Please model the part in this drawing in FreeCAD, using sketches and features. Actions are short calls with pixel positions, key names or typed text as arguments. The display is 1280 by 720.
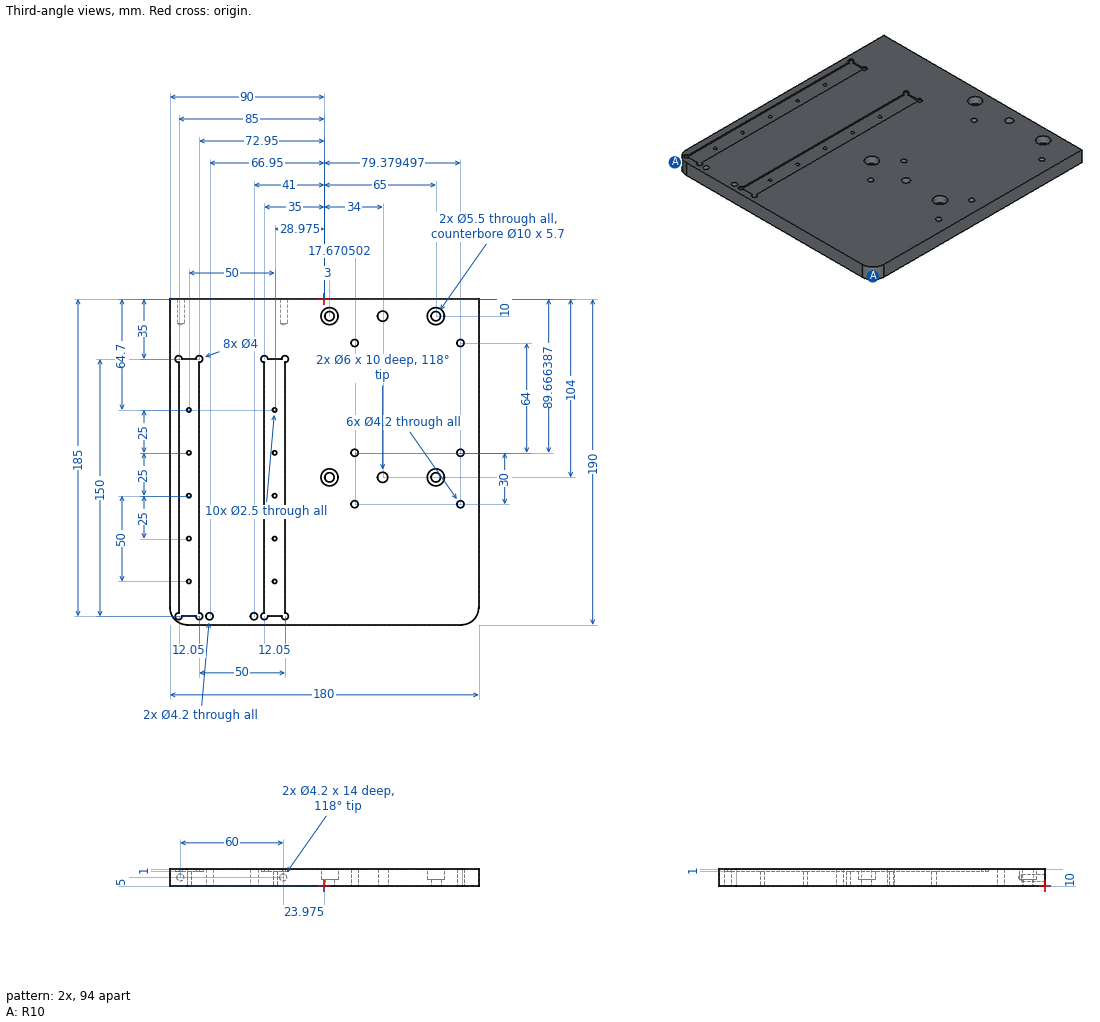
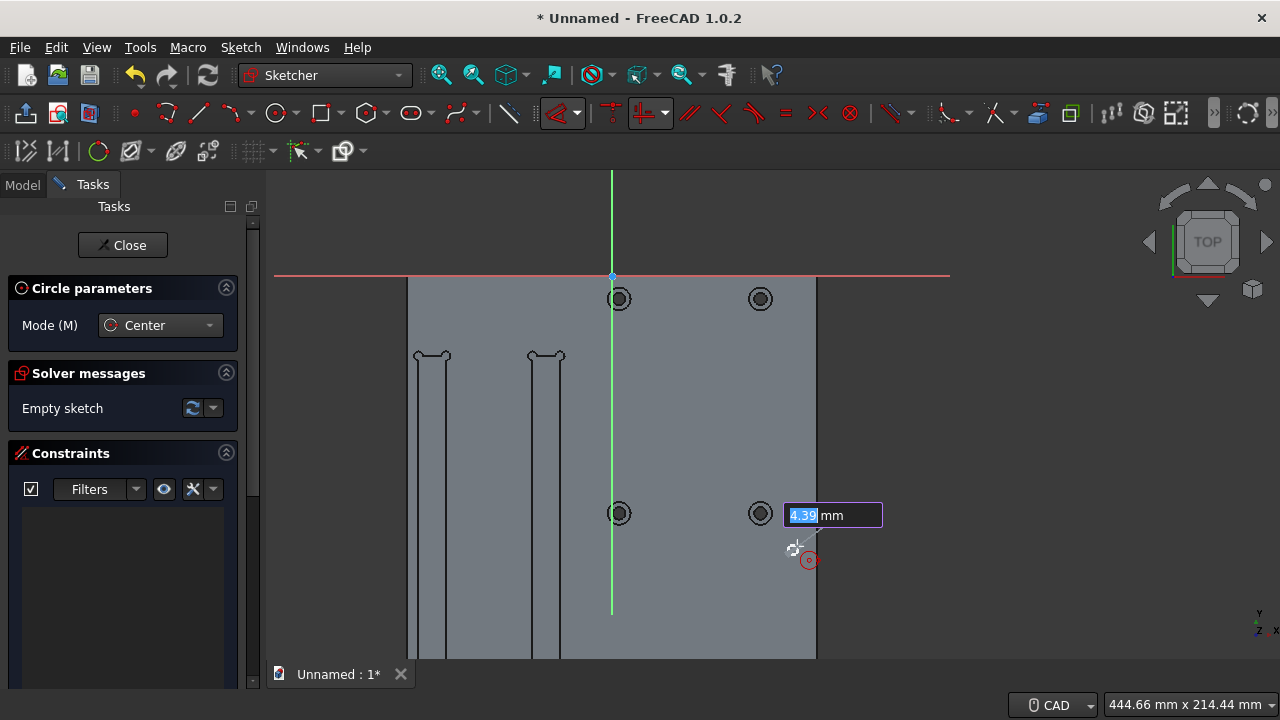
text(4.2)
key(Return)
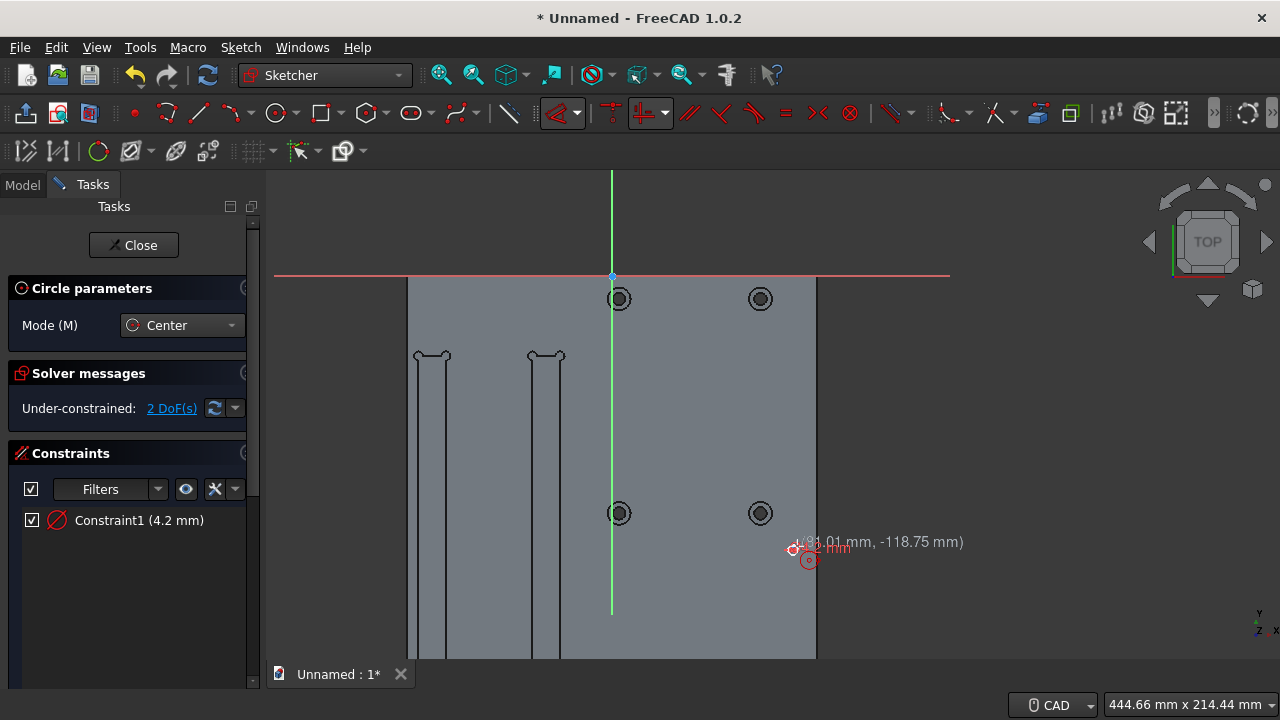
scroll(653, 549, up, 8)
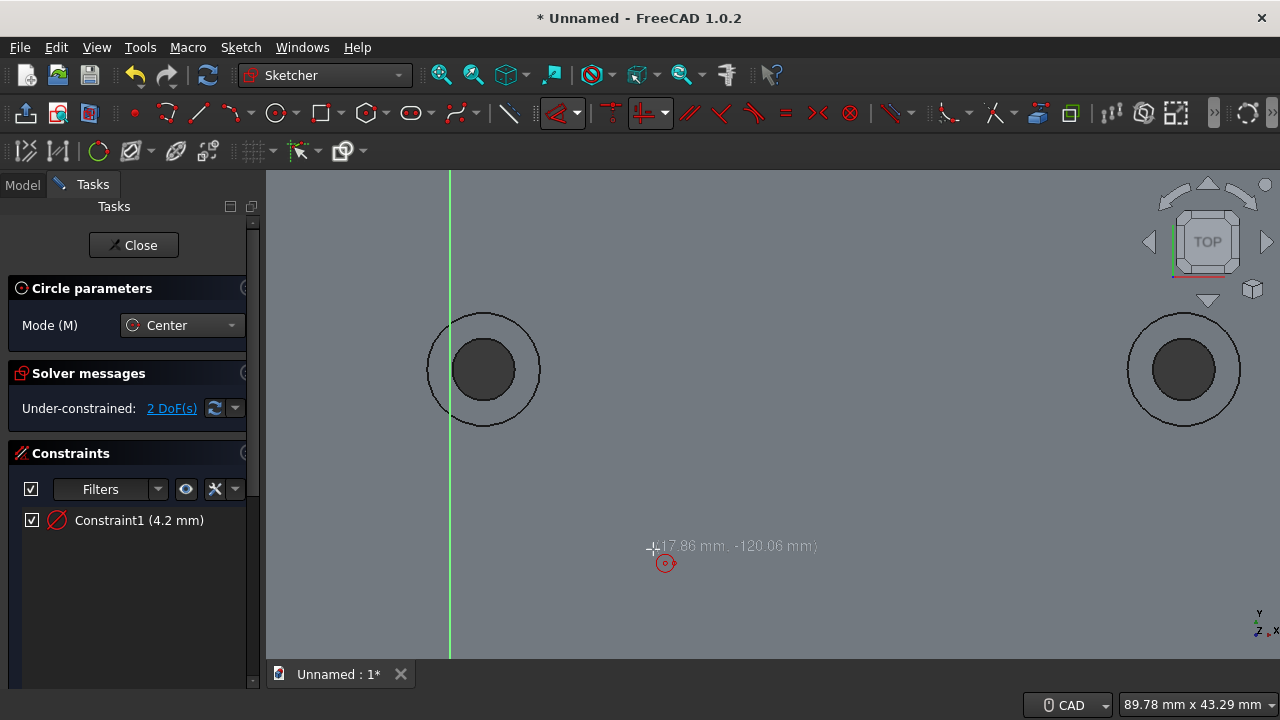
scroll(653, 549, down, 8)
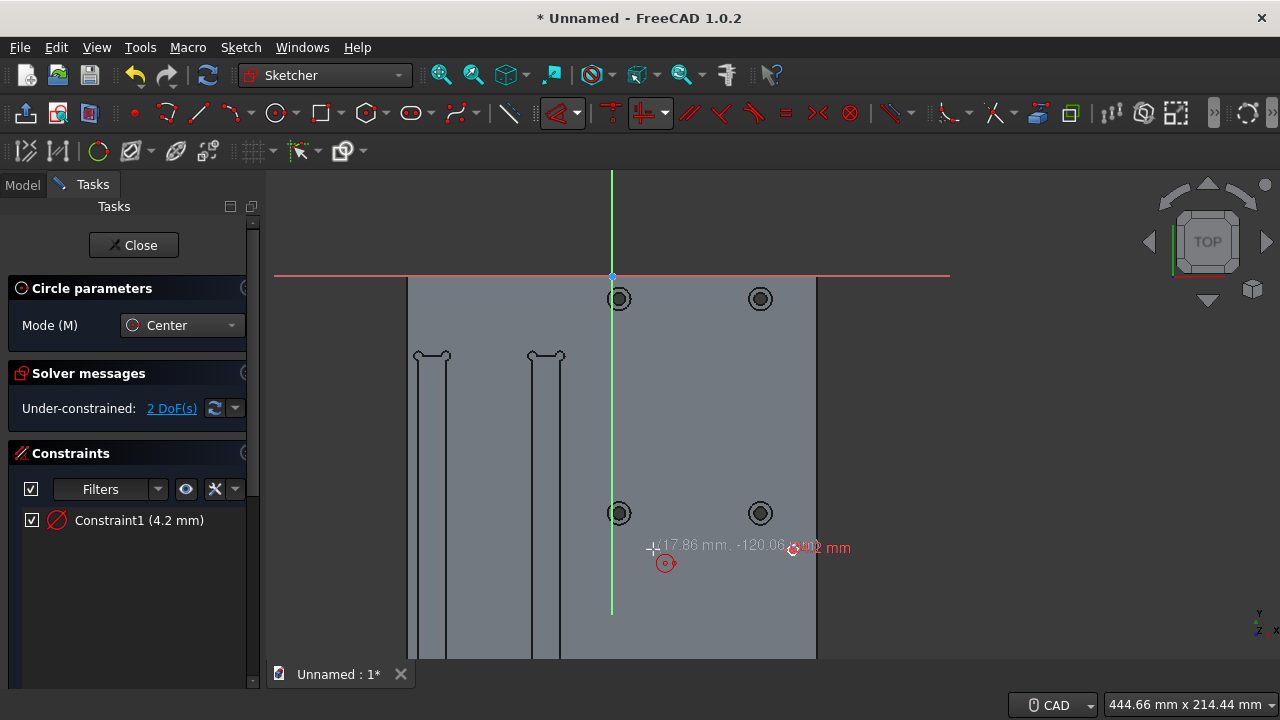
click(653, 549)
move(656, 546)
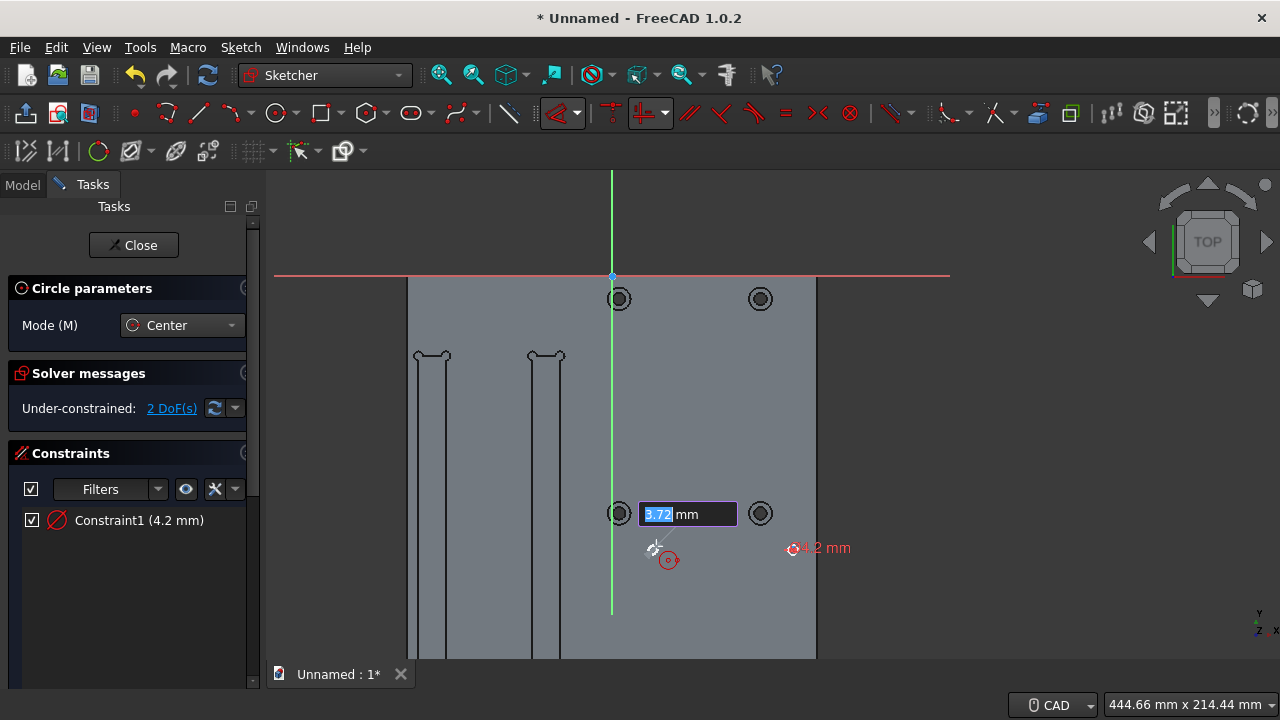
text(4.2)
key(Return)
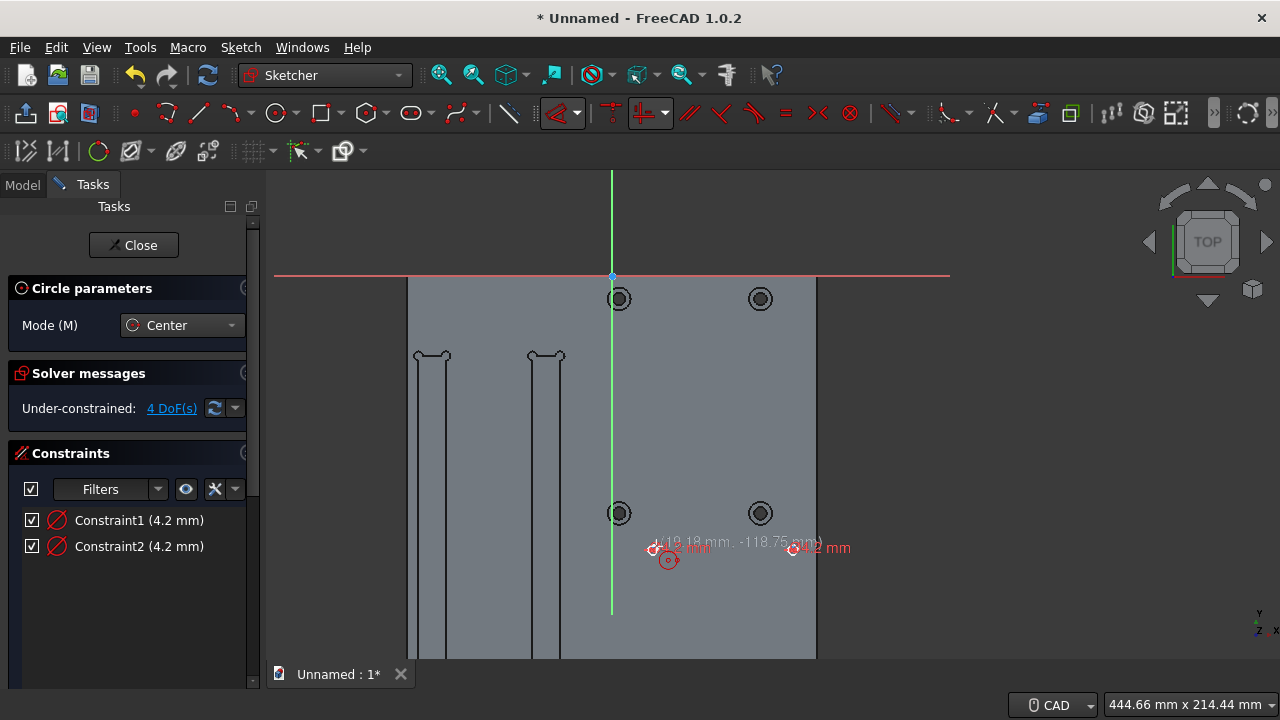
scroll(653, 481, up, 8)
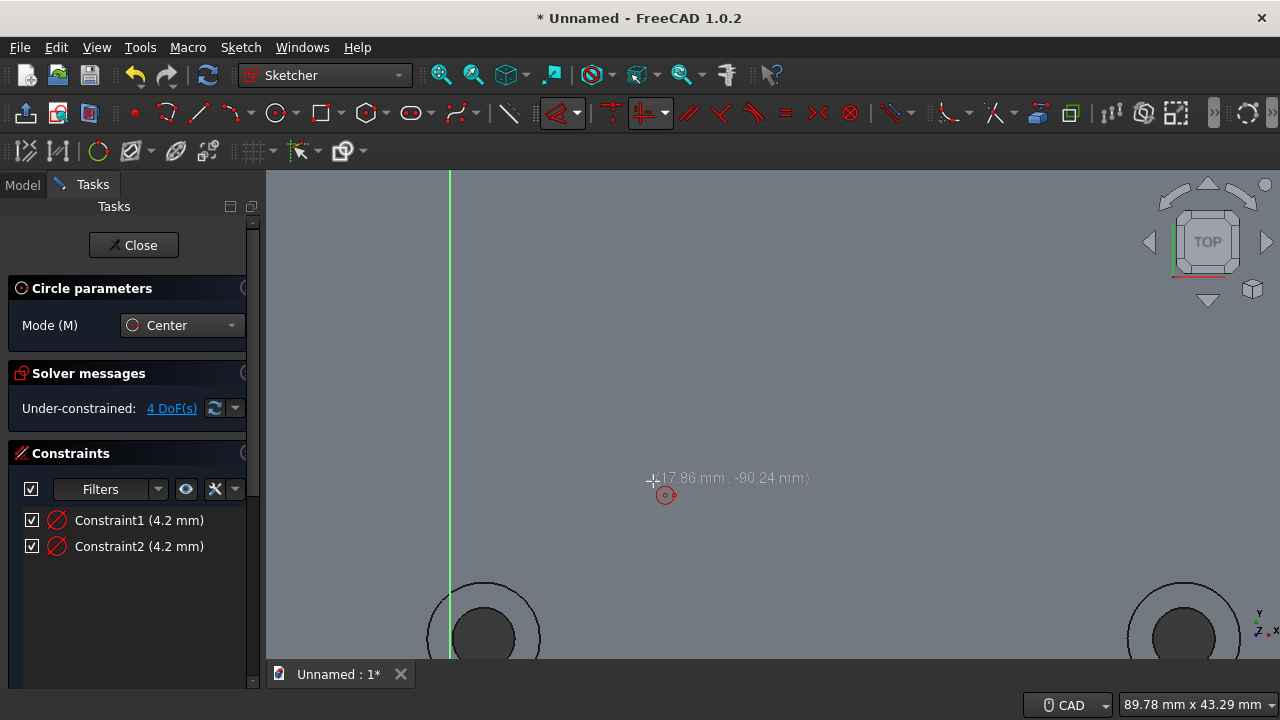
scroll(653, 481, down, 8)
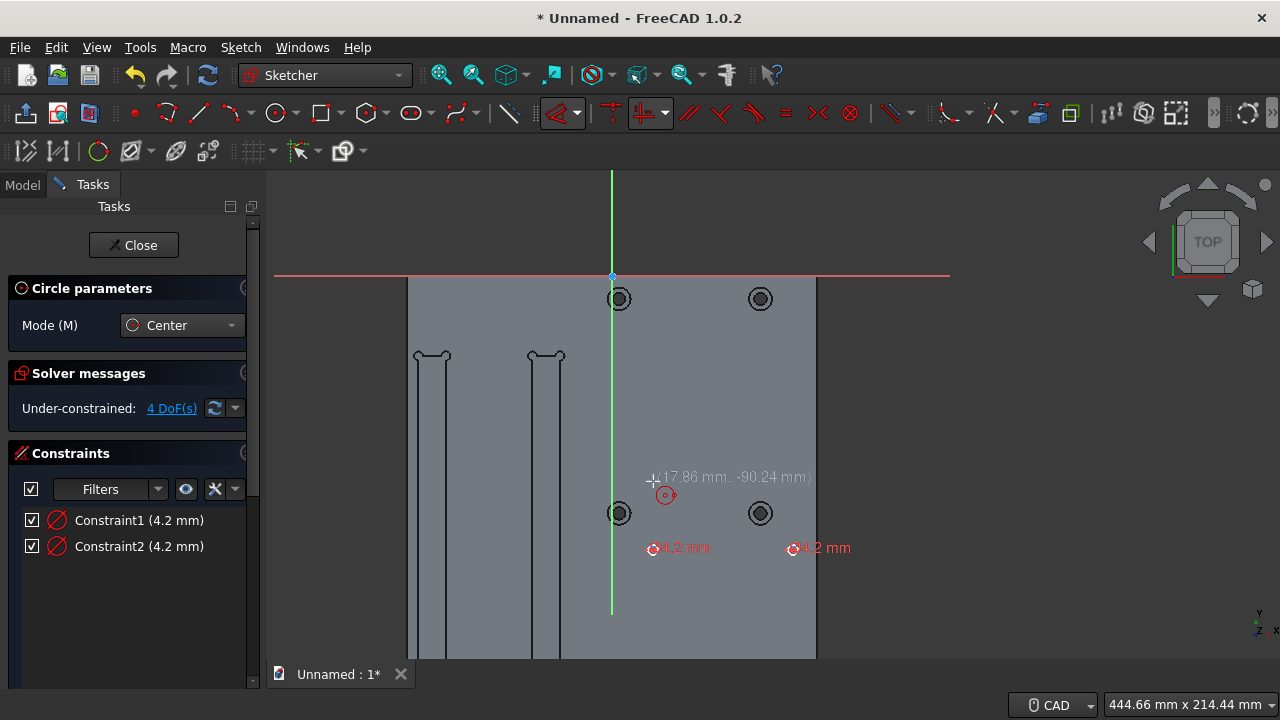
click(653, 481)
move(656, 477)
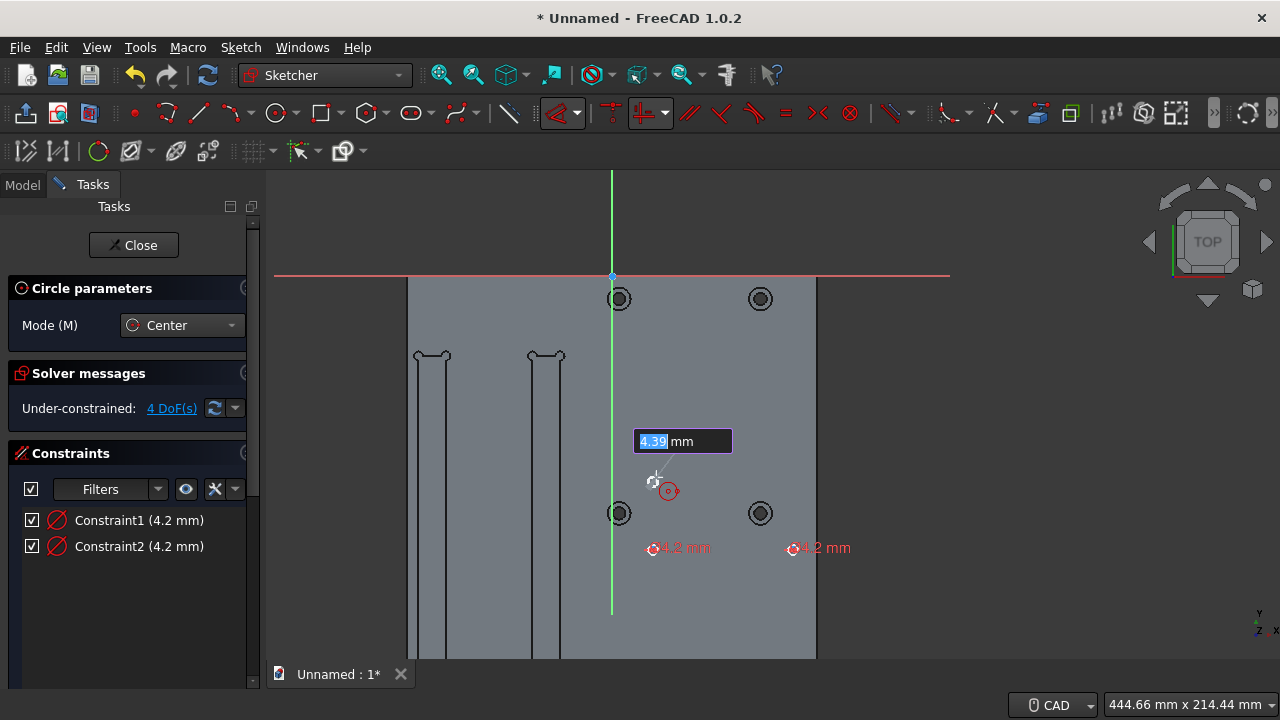
text(4.2)
key(Return)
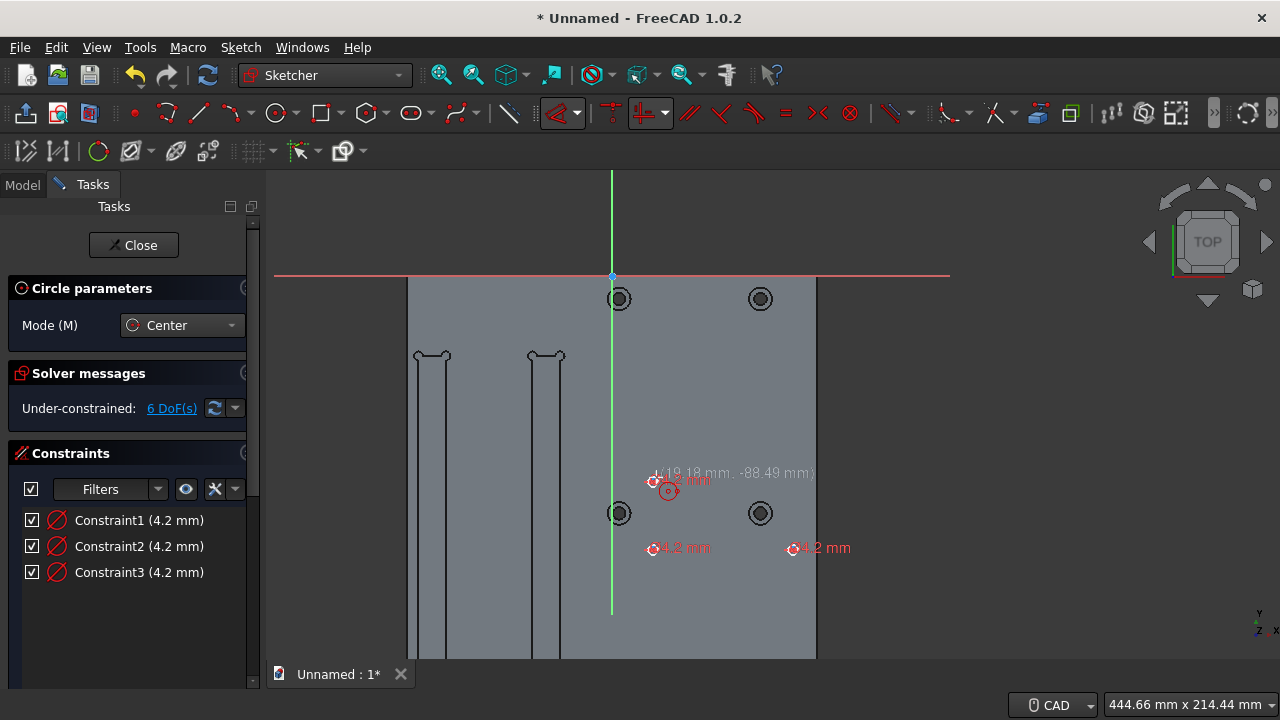
scroll(793, 481, up, 8)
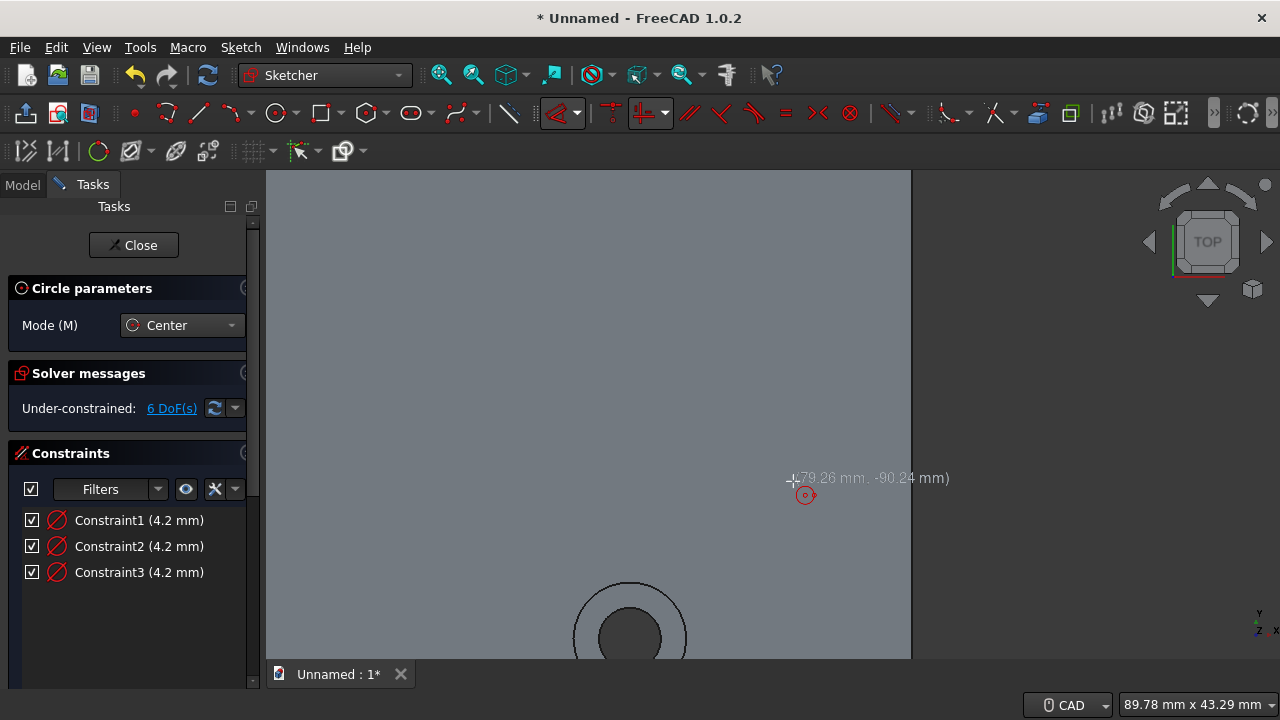
scroll(793, 481, down, 8)